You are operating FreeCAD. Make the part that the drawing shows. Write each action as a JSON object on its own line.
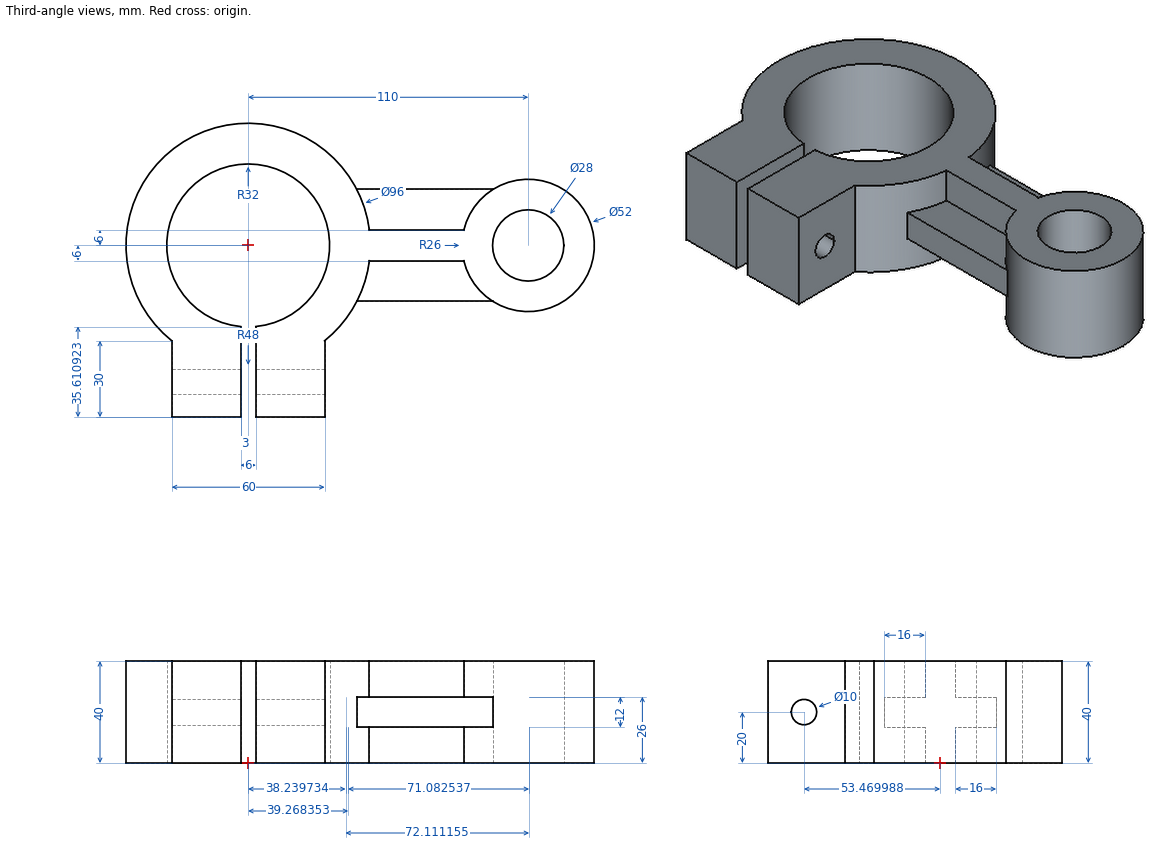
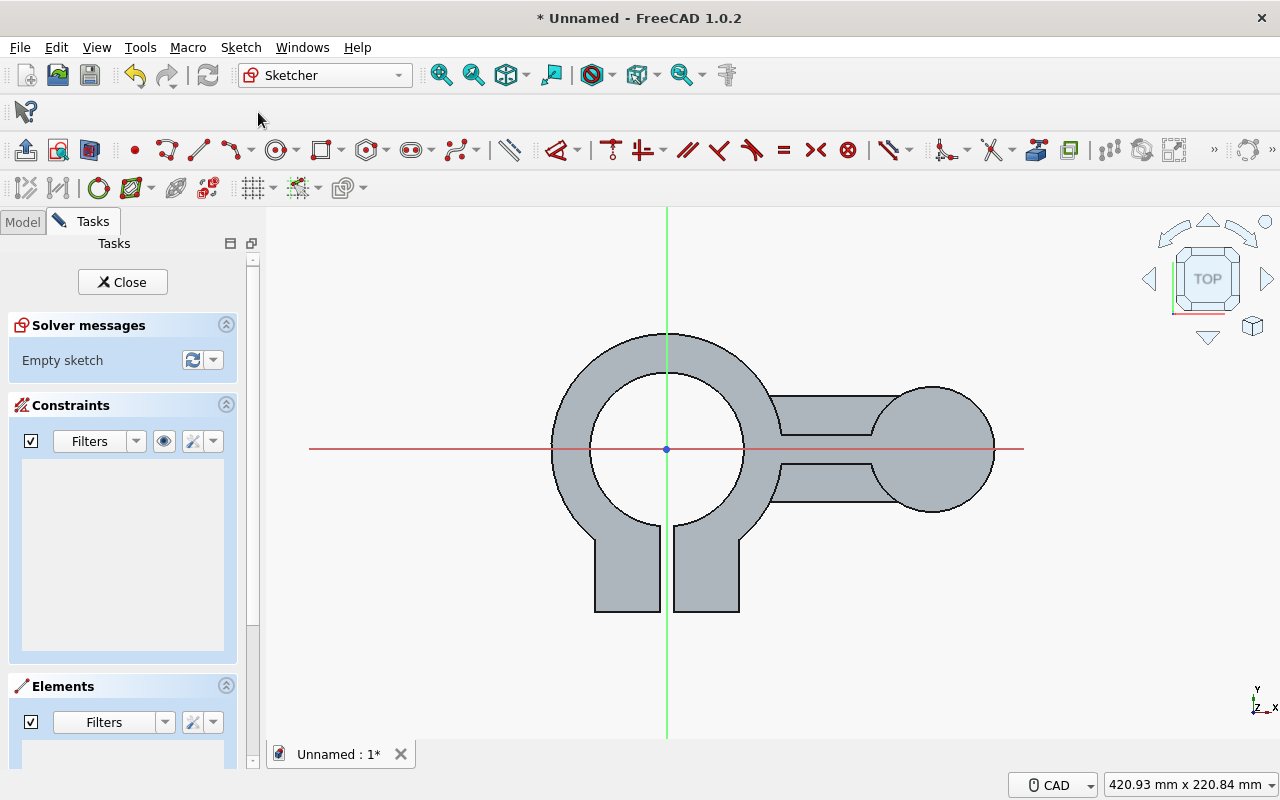
{"action": "scroll", "coordinate": [990, 444], "scroll_direction": "up", "scroll_amount": 8}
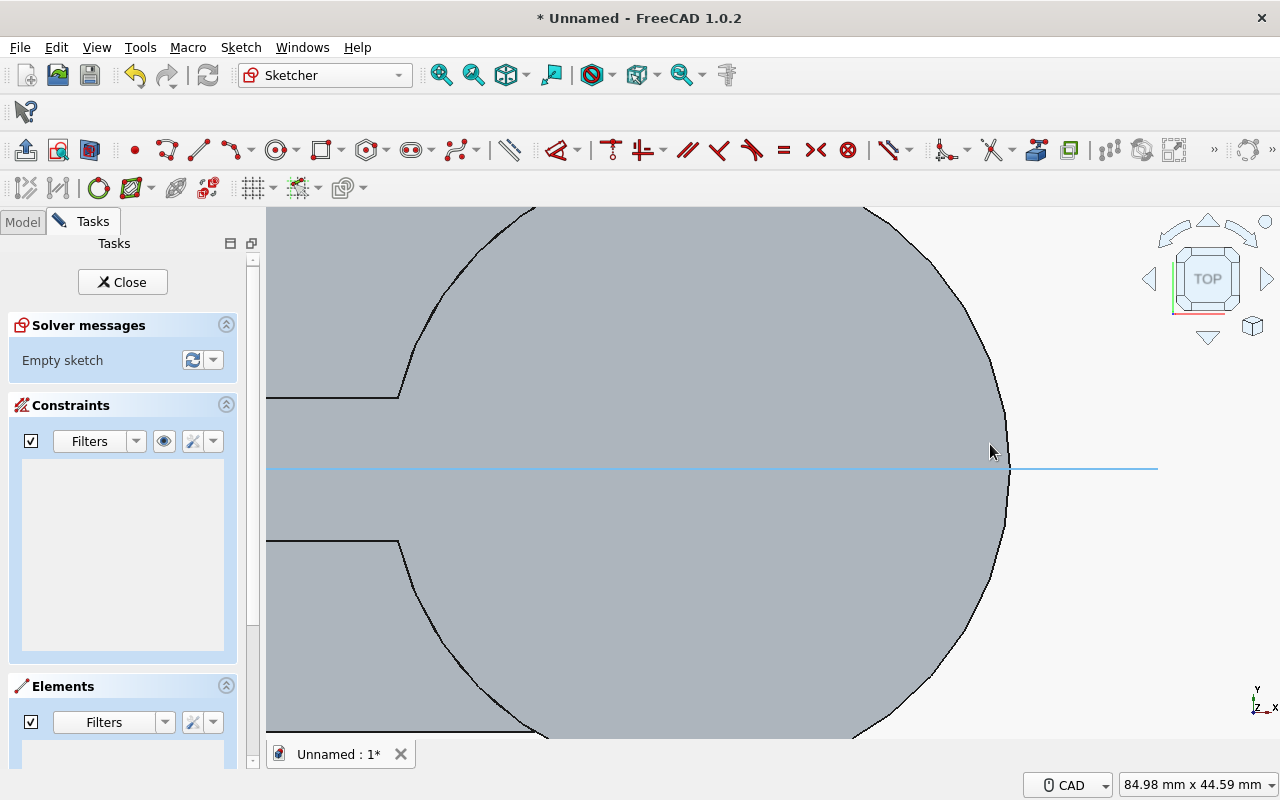
{"action": "left_click", "coordinate": [276, 150]}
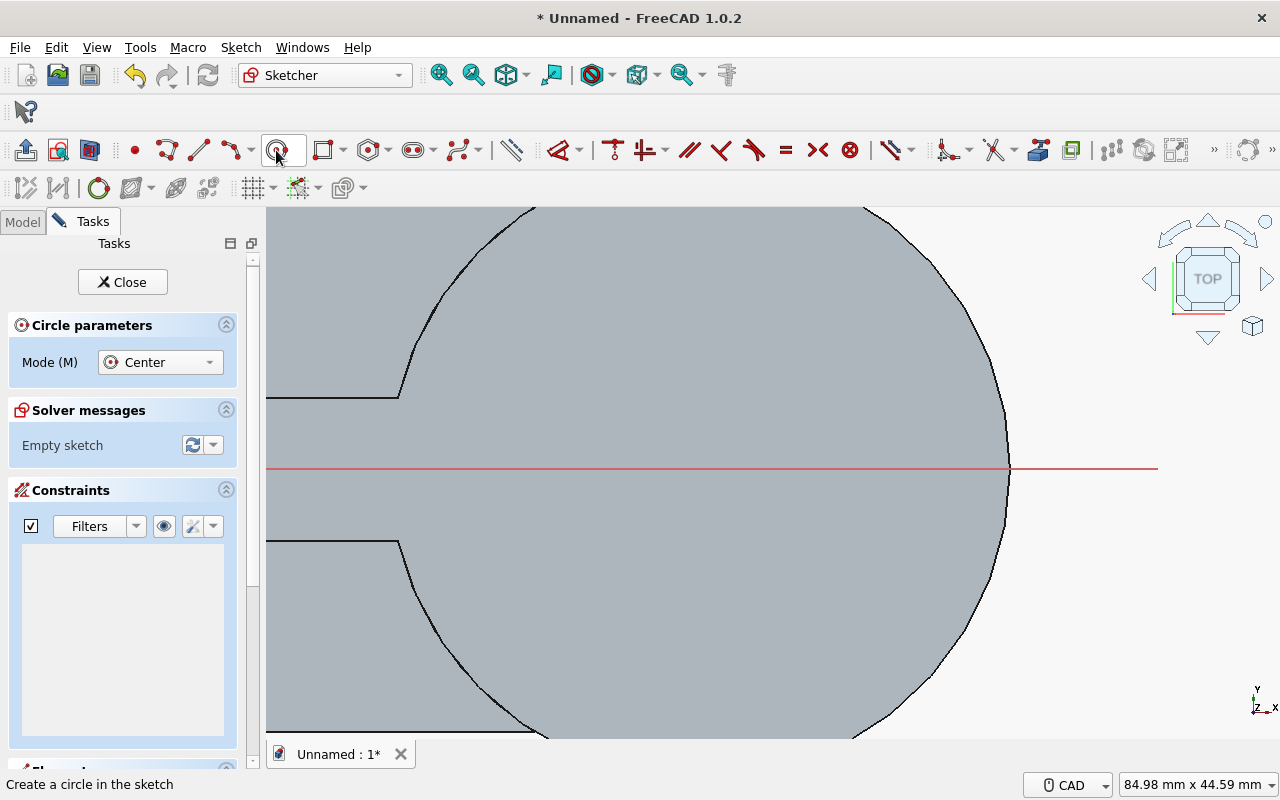
{"action": "left_click", "coordinate": [700, 469]}
{"action": "left_click", "coordinate": [818, 351]}
{"action": "key", "text": "Escape"}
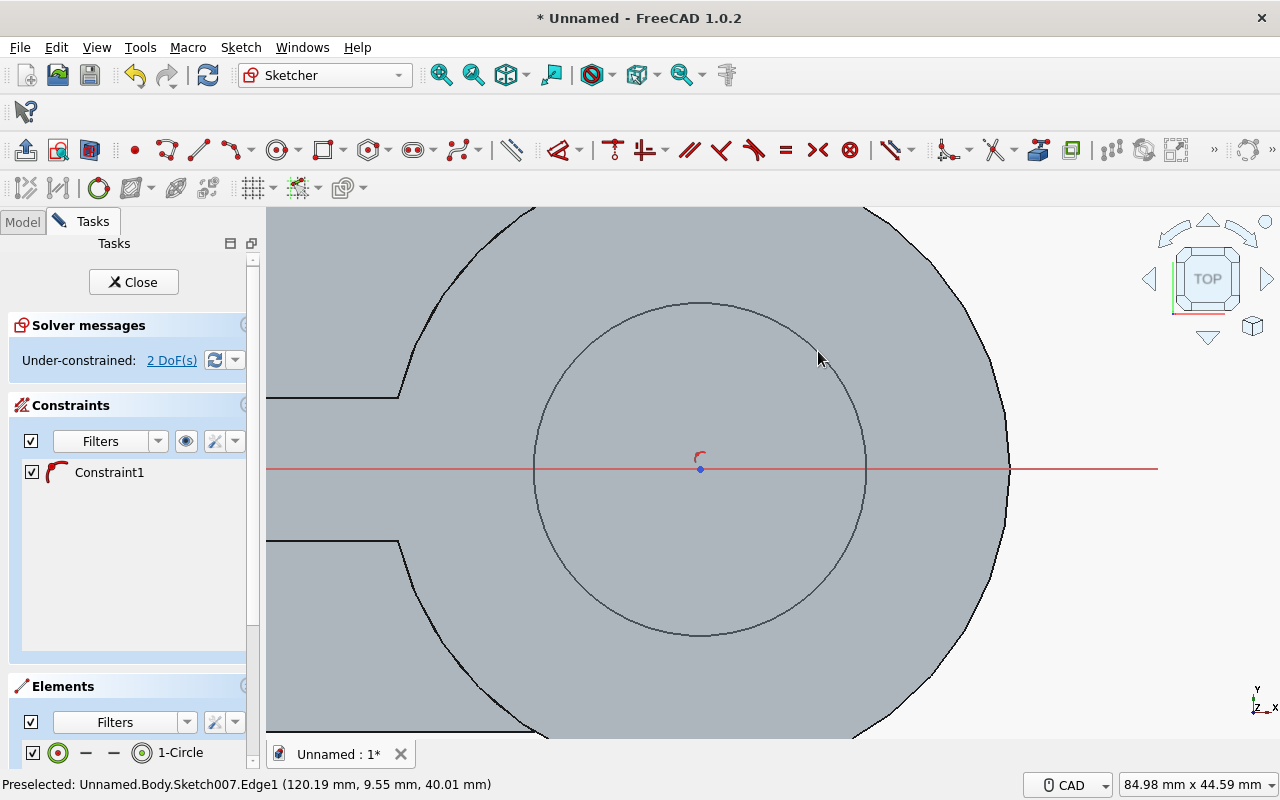
{"action": "left_click", "coordinate": [558, 150]}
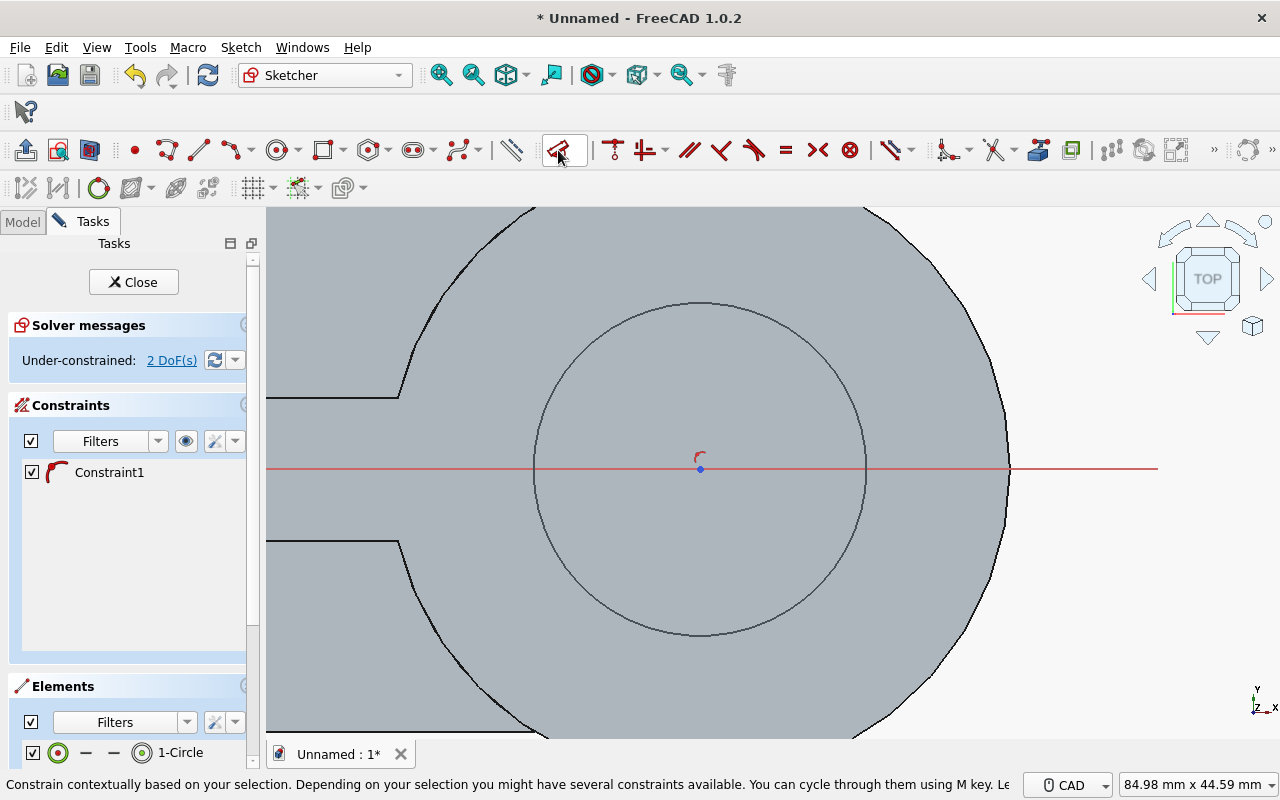
{"action": "left_click", "coordinate": [817, 351]}
{"action": "left_click", "coordinate": [839, 328]}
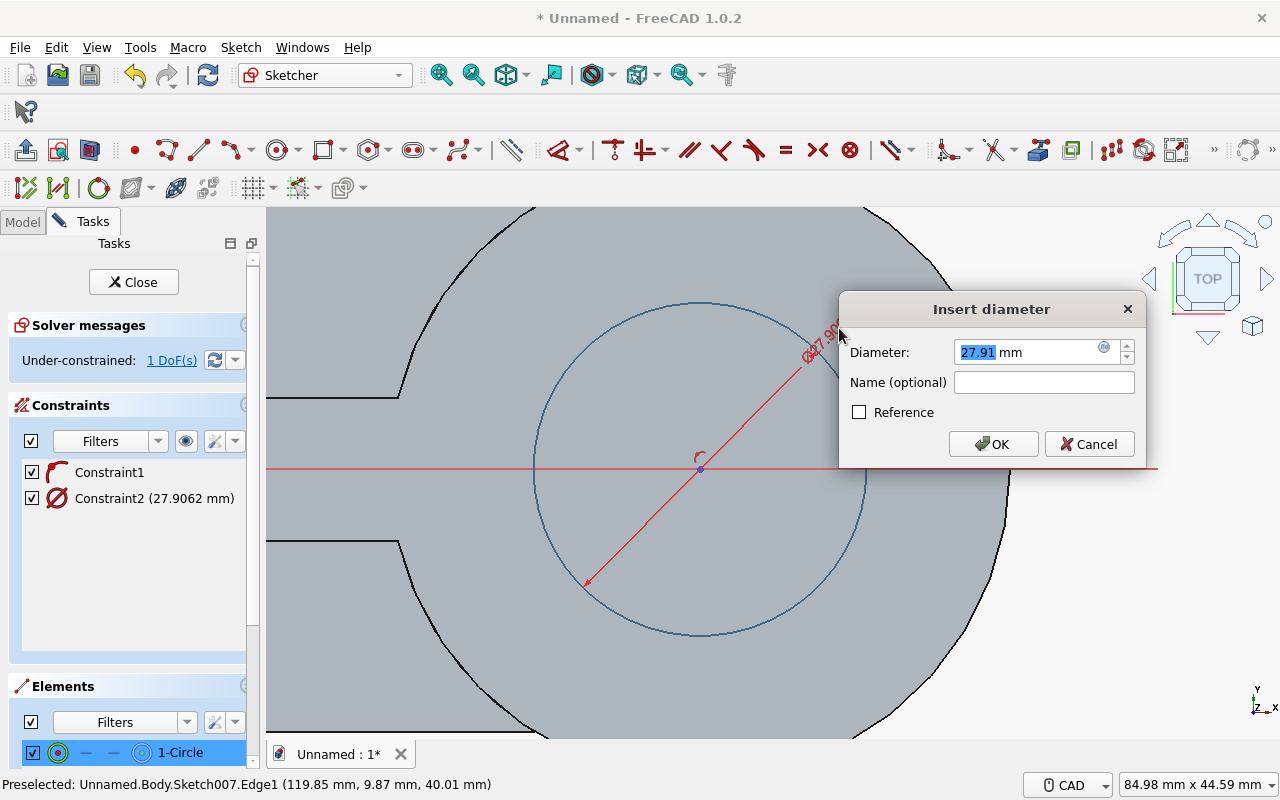
{"action": "type", "text": "28"}
{"action": "key", "text": "Return"}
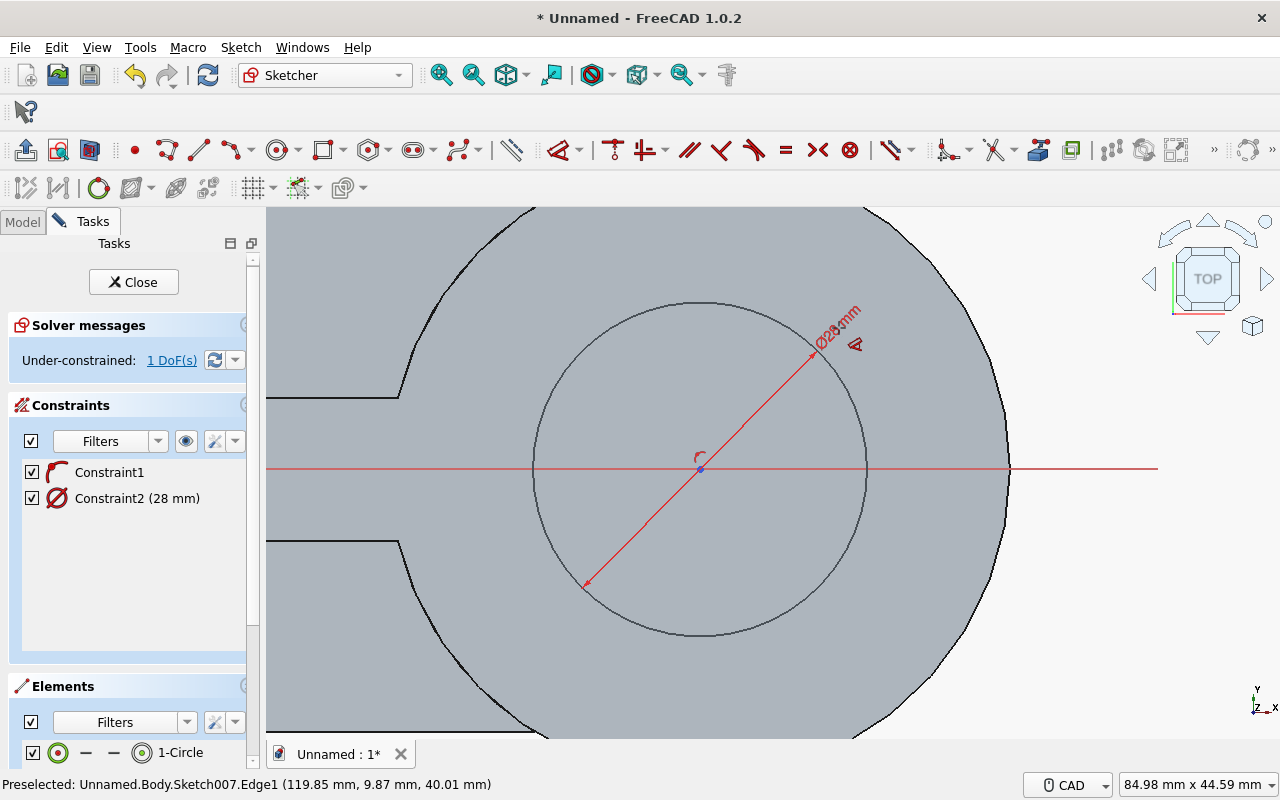
{"action": "left_click", "coordinate": [700, 469]}
{"action": "left_click", "coordinate": [497, 503]}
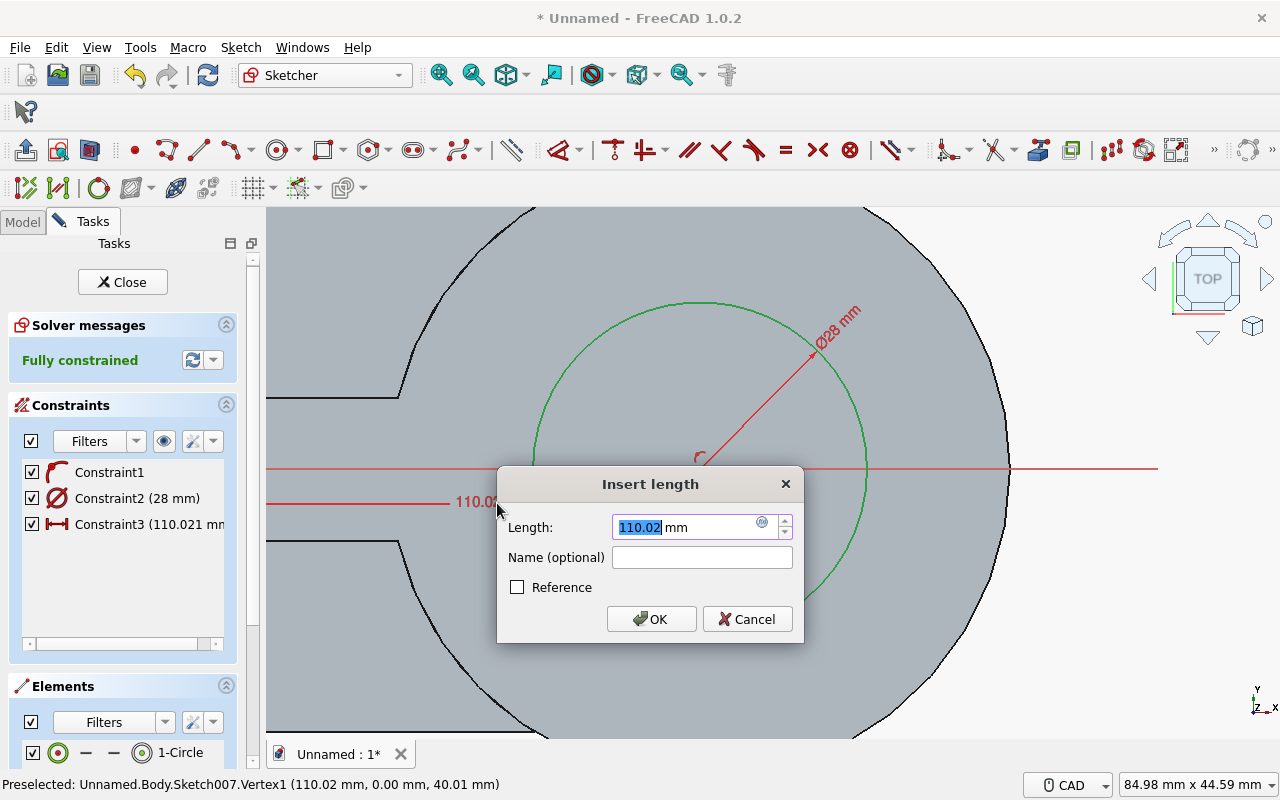
{"action": "type", "text": "110"}
{"action": "key", "text": "Return"}
{"action": "key", "text": "Escape"}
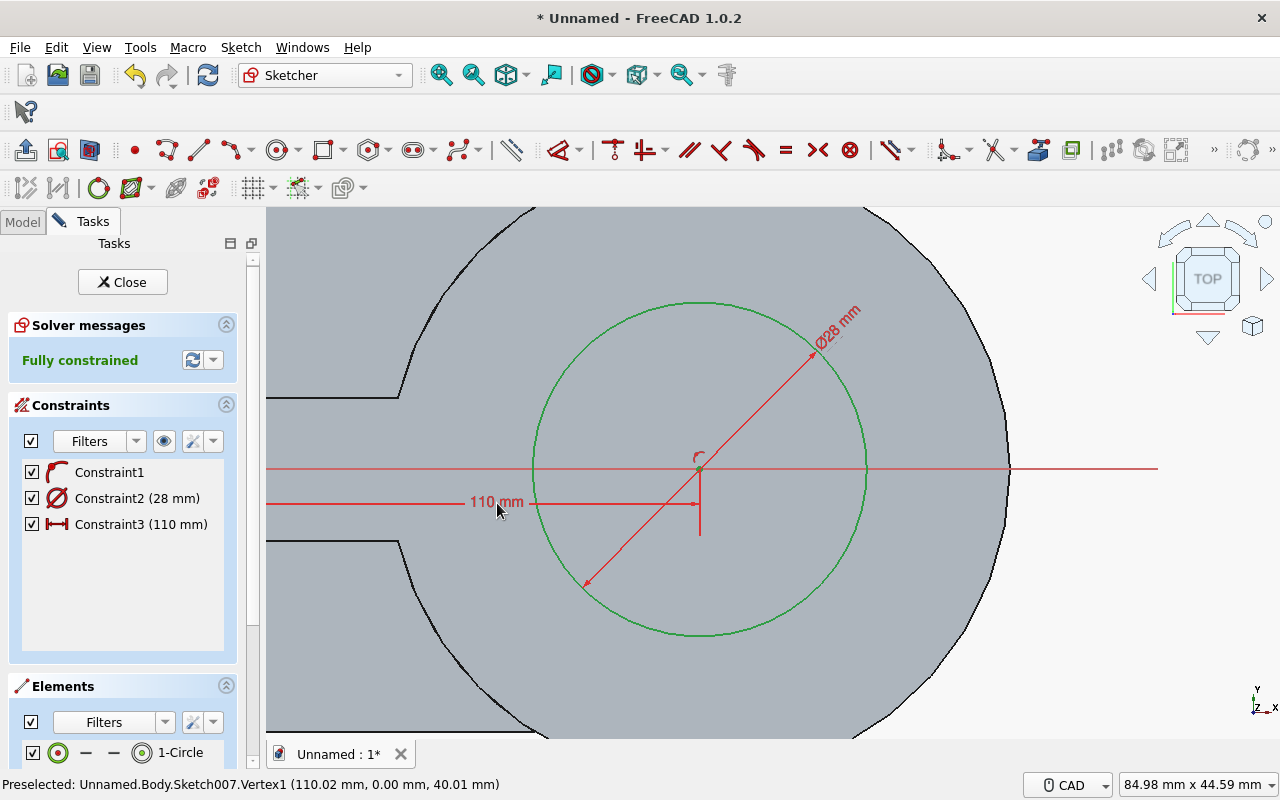
{"action": "left_click", "coordinate": [123, 282]}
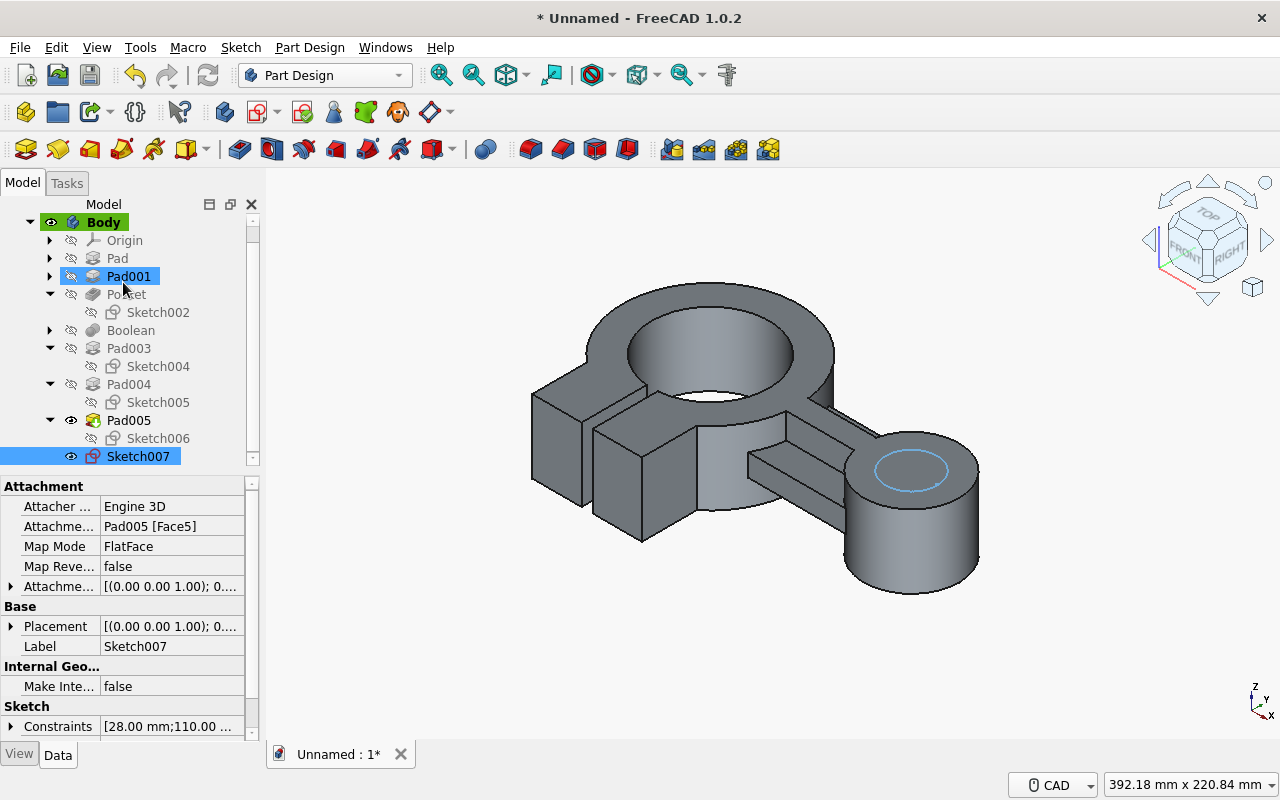
{"action": "left_click", "coordinate": [240, 150]}